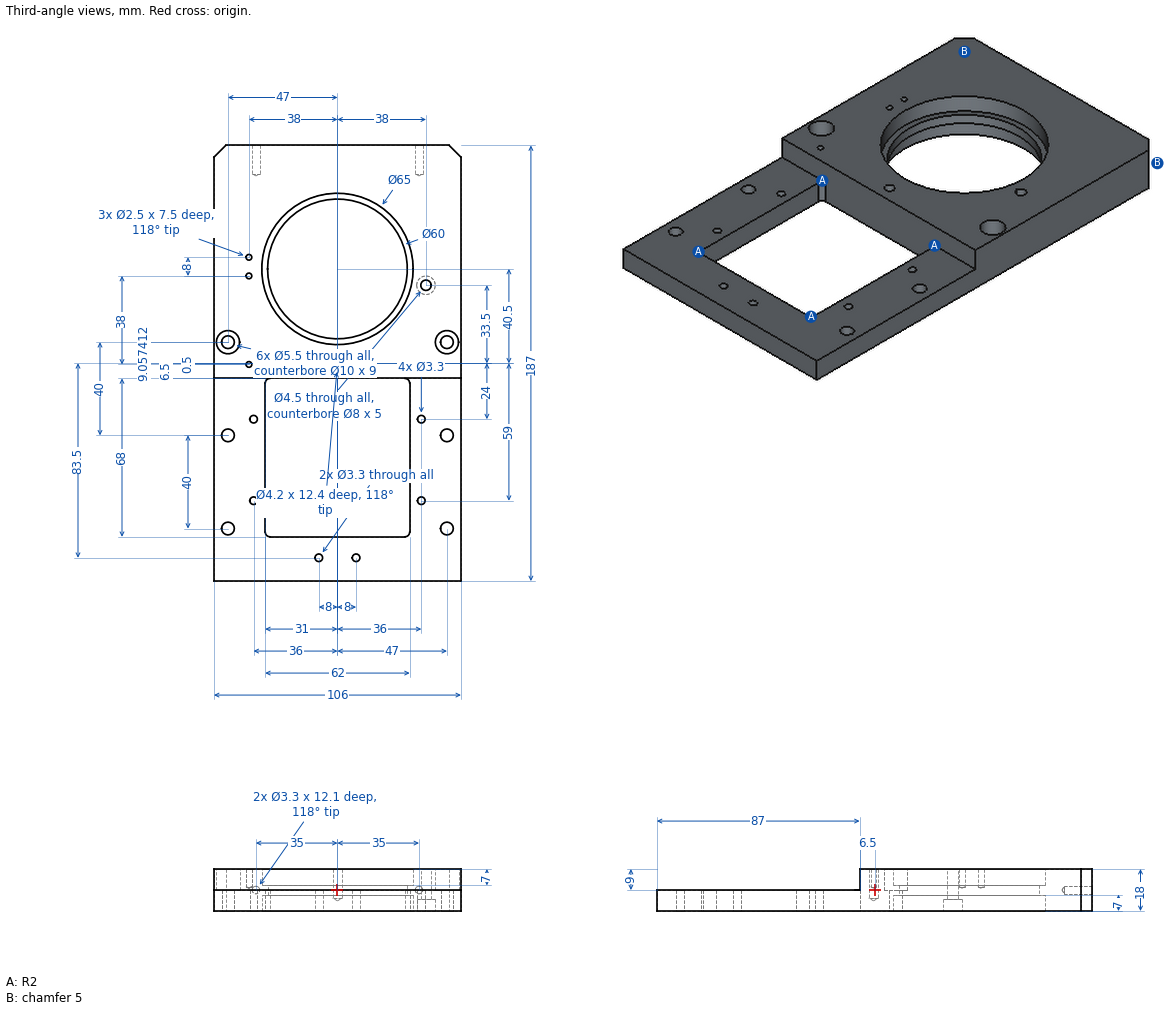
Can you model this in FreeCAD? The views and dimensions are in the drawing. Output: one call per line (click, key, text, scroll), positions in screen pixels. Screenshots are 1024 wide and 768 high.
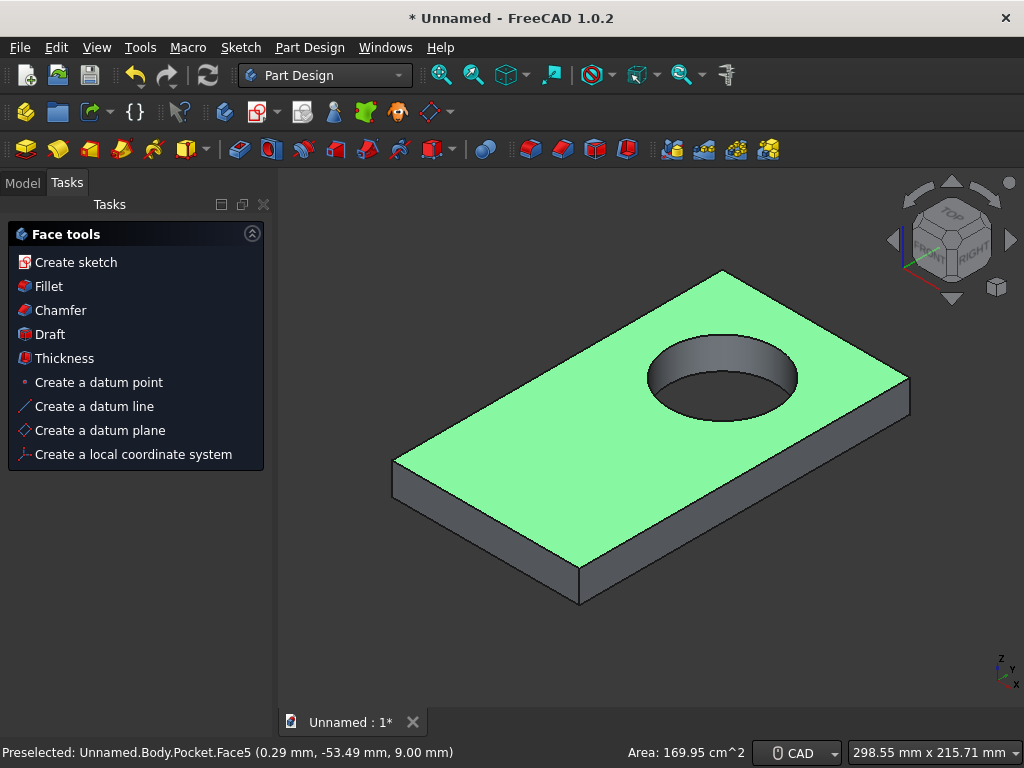
click(258, 112)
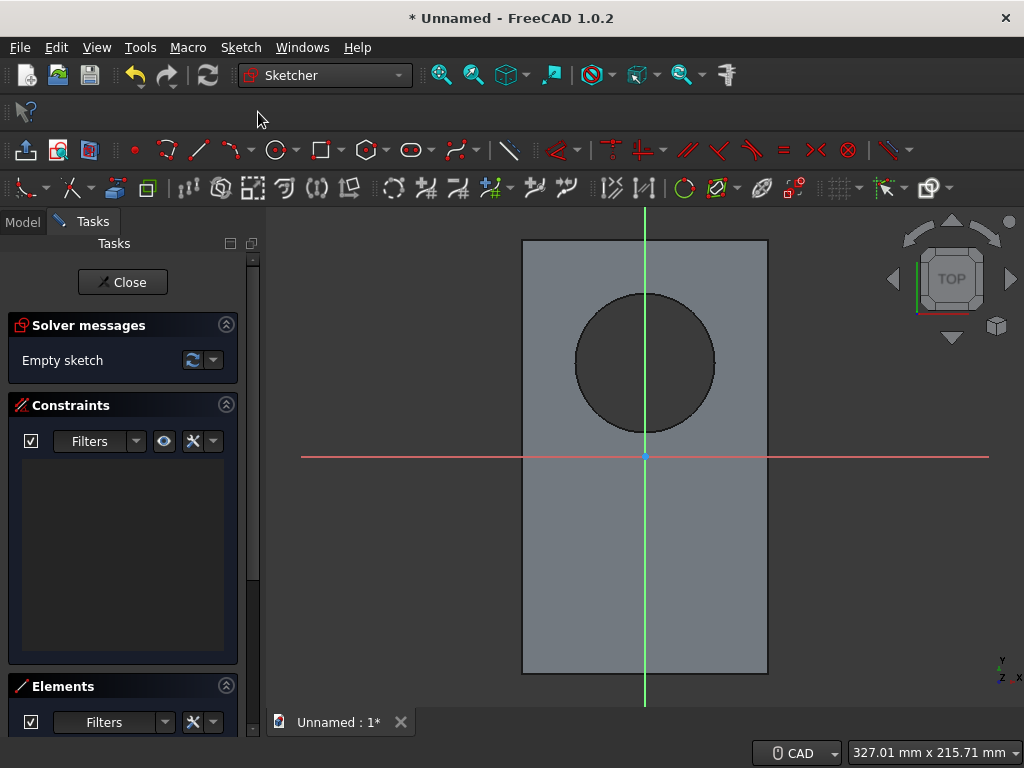
scroll(728, 269, up, 3)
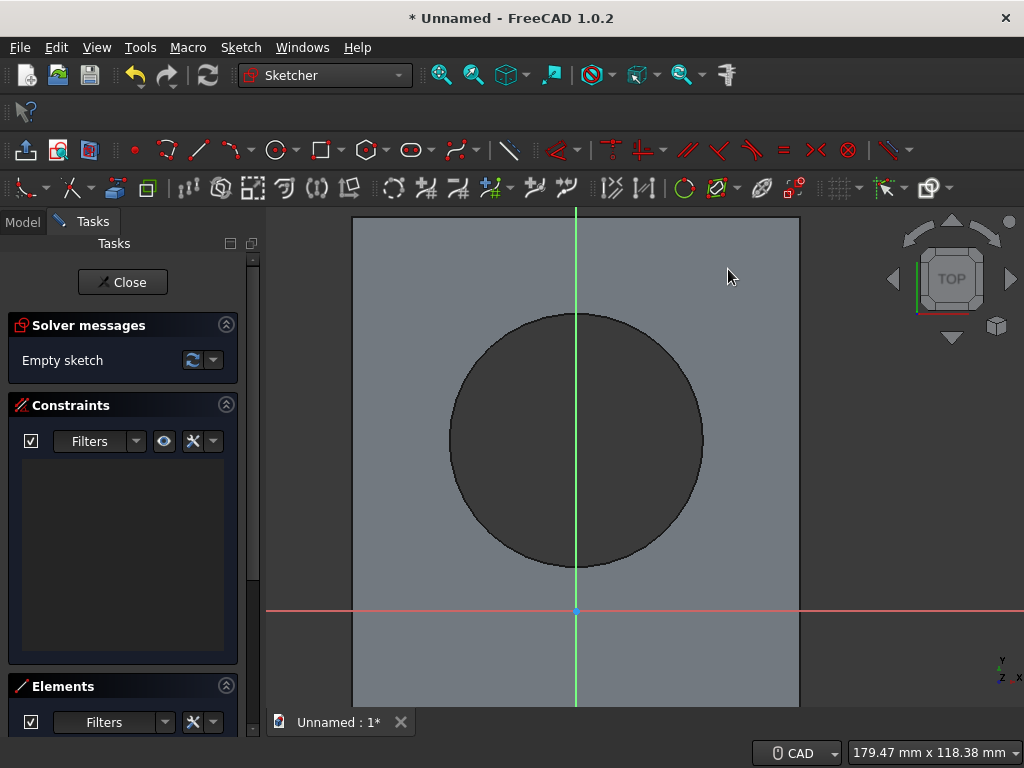
click(276, 150)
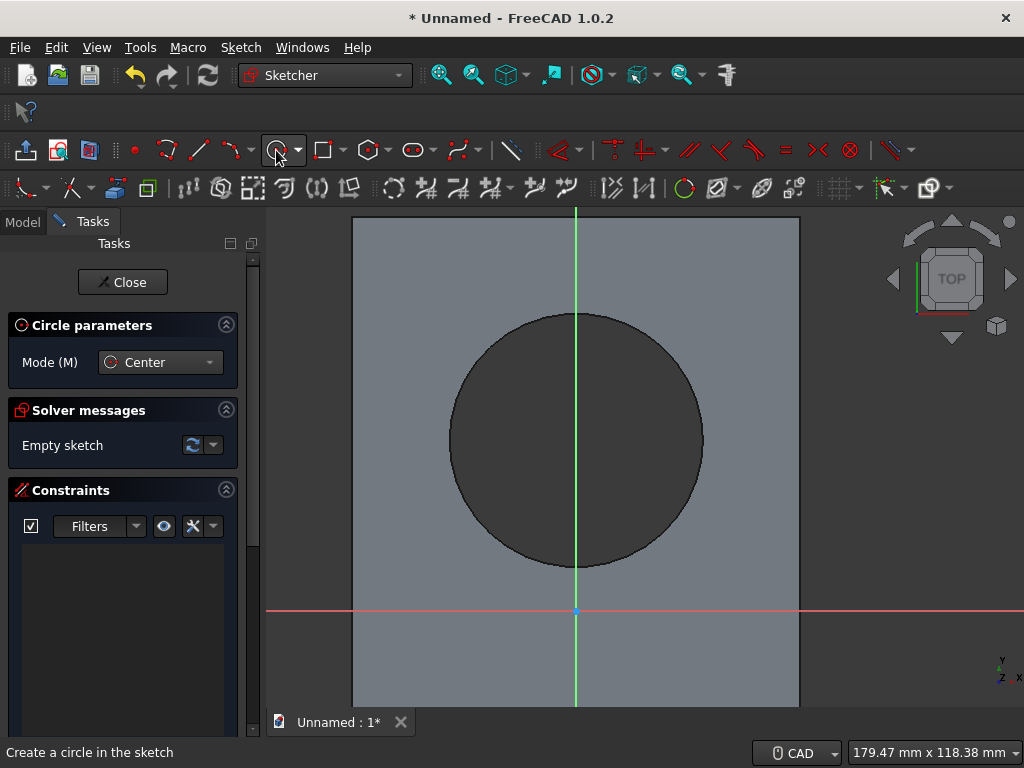
click(576, 440)
click(673, 343)
key(Escape)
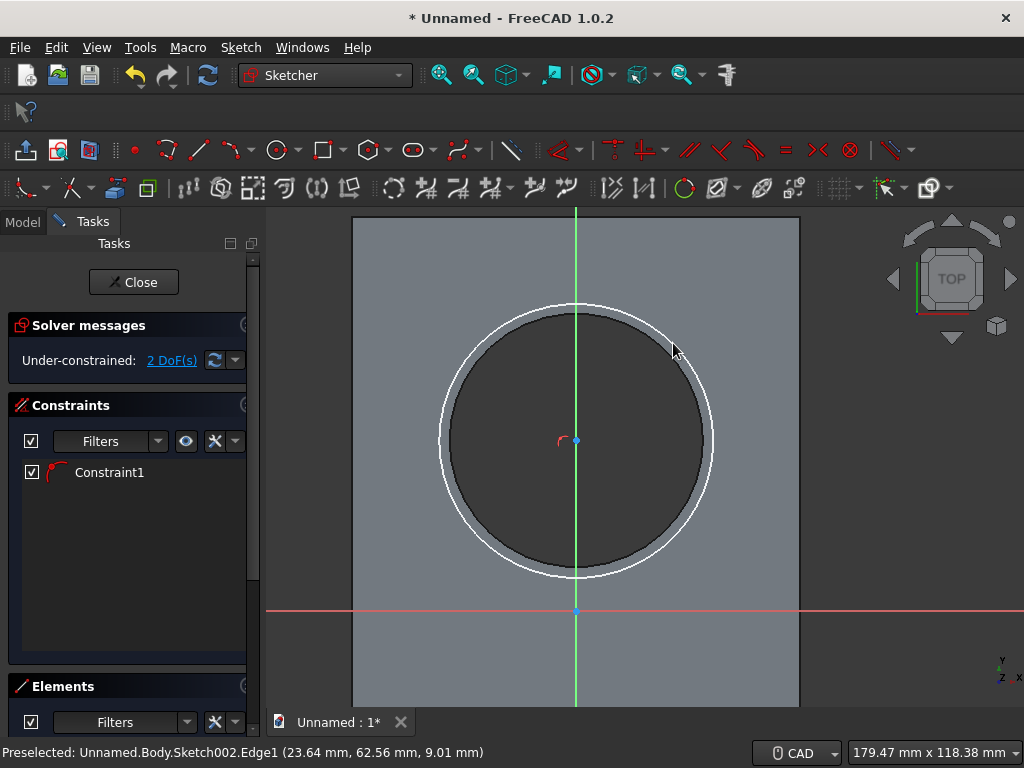
click(558, 150)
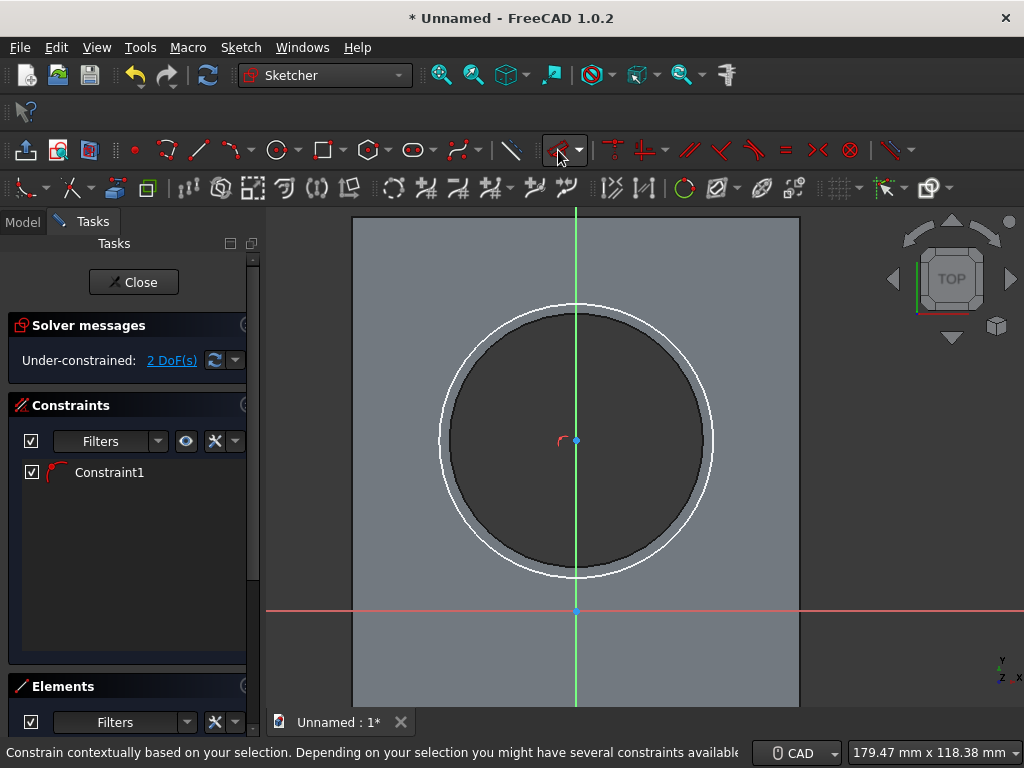
click(673, 344)
click(696, 321)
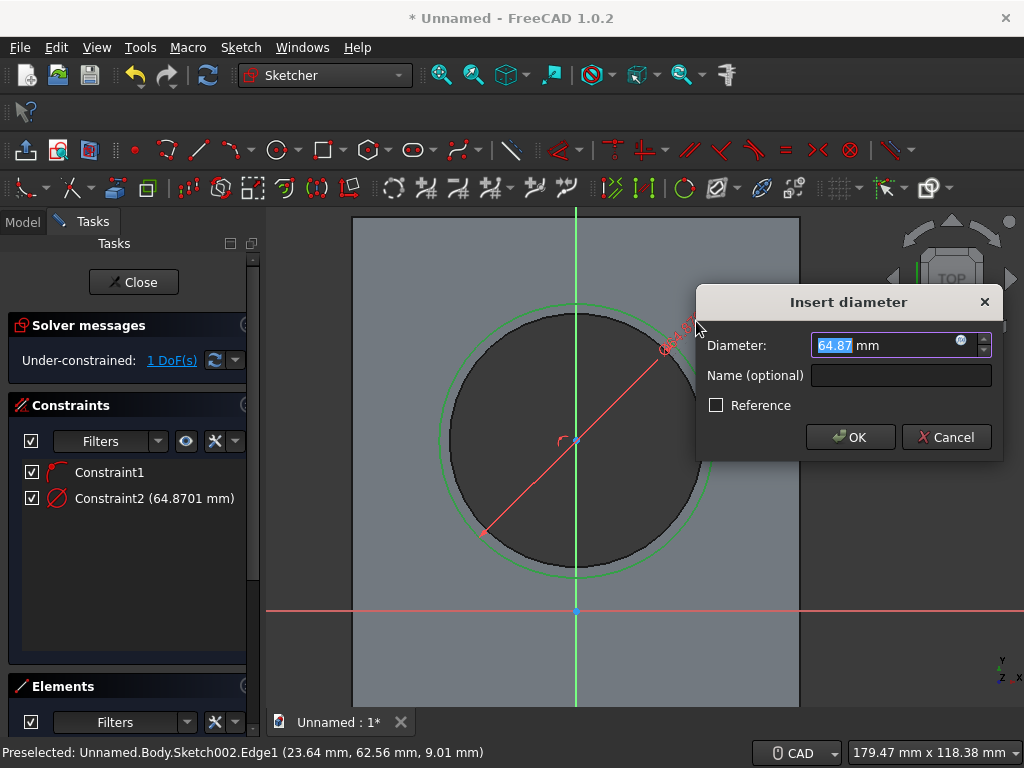
text(65)
key(Return)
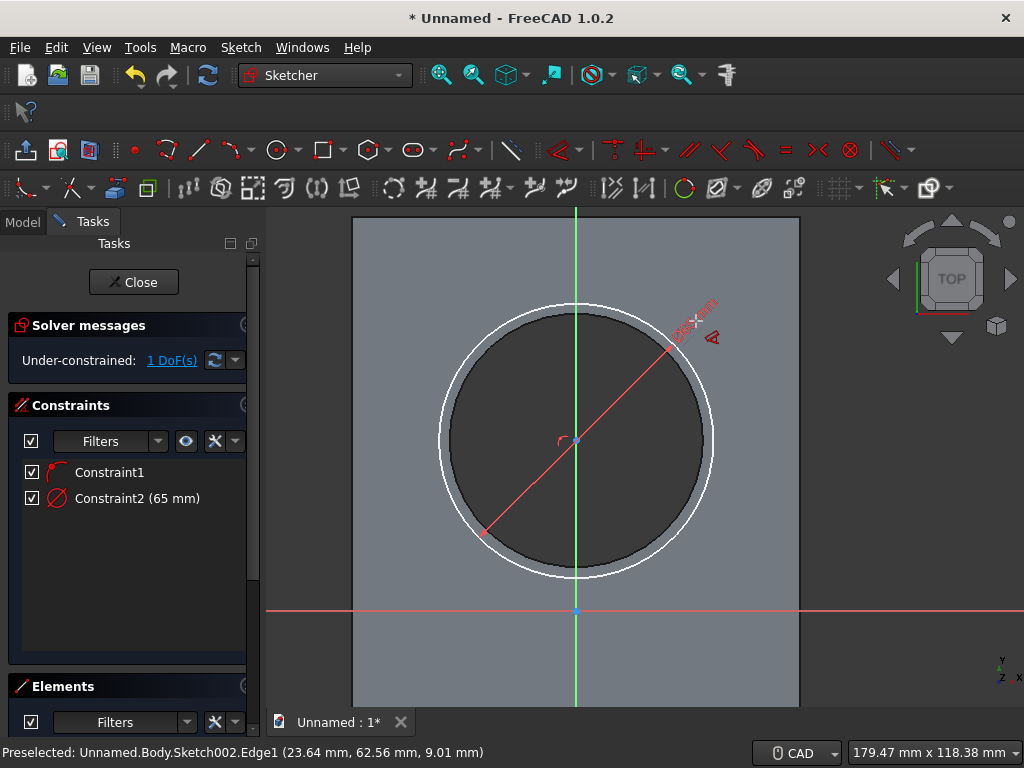
click(576, 441)
click(610, 526)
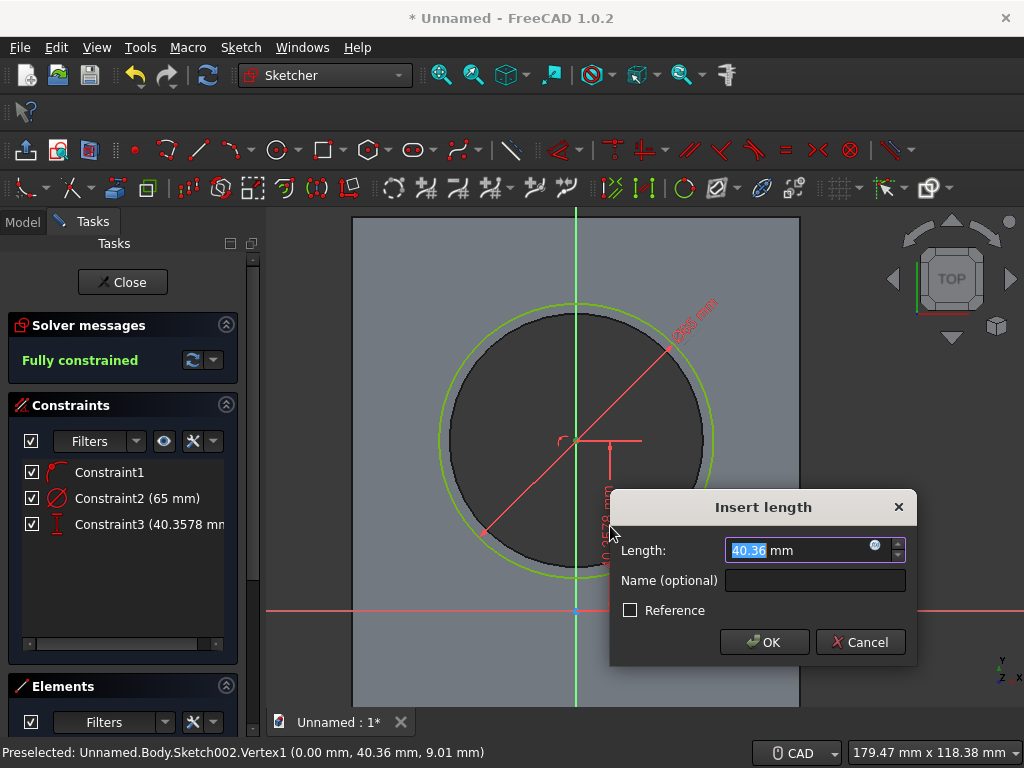
text(40.5)
key(Return)
key(Escape)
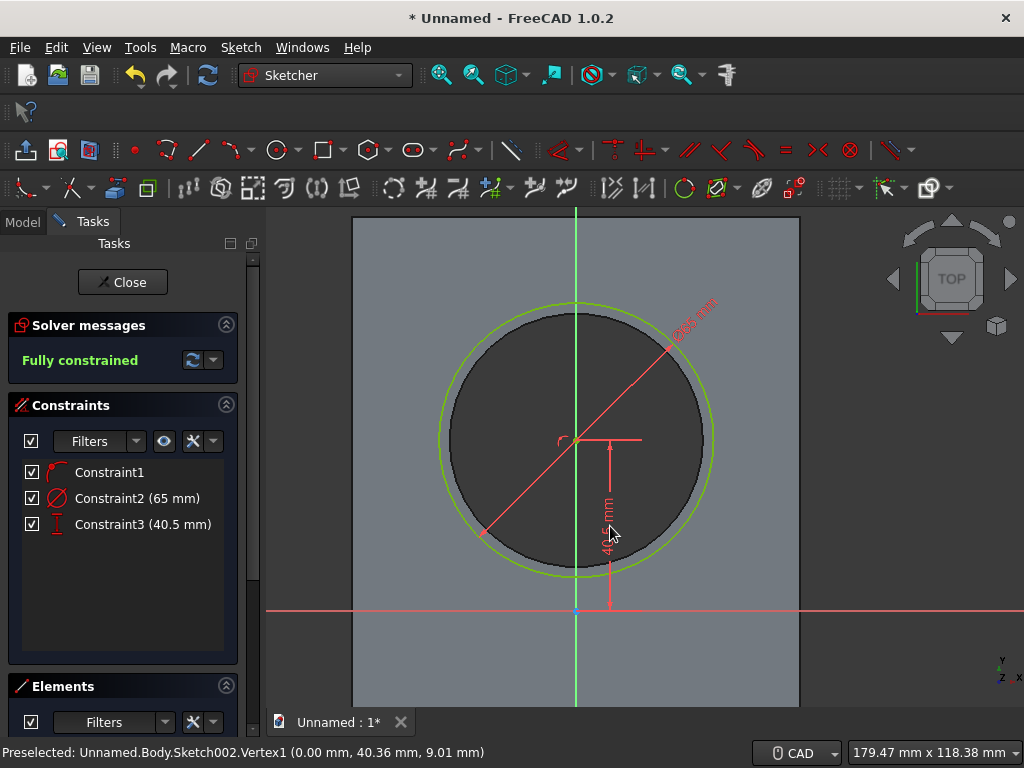
click(123, 282)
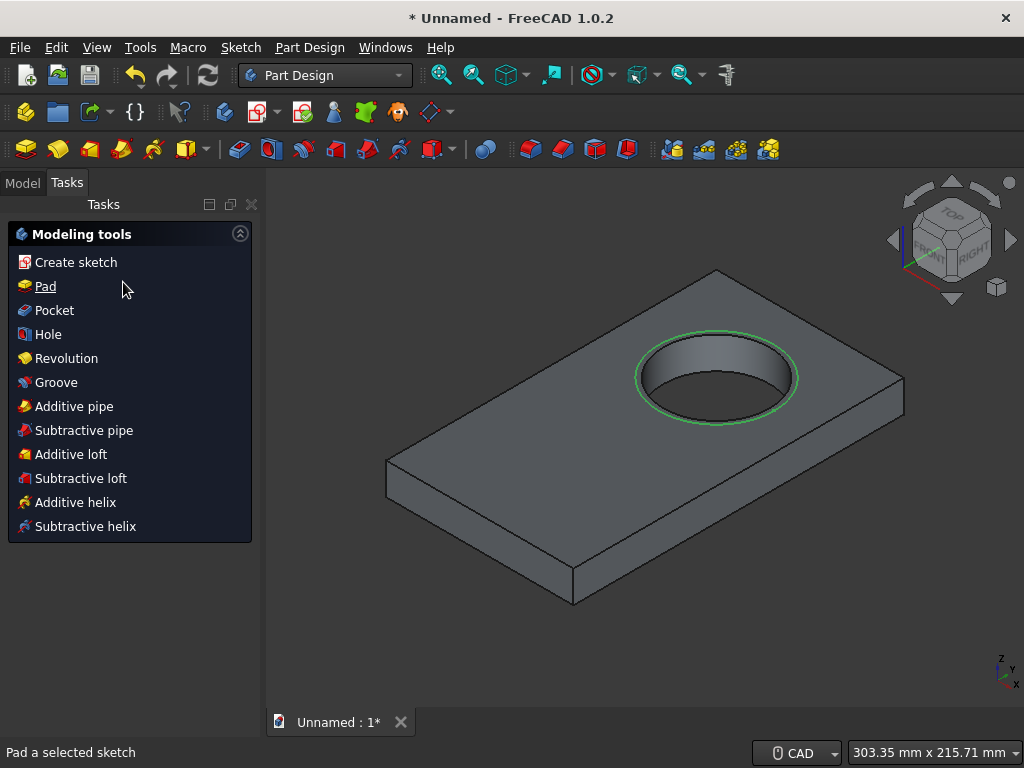
click(240, 150)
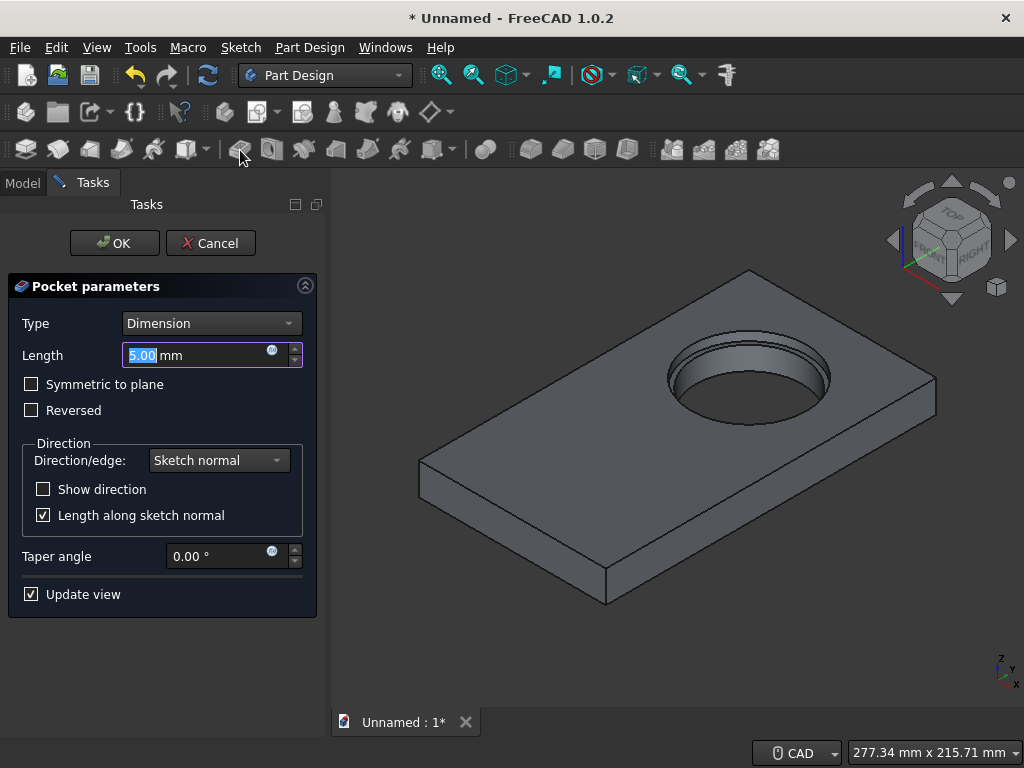
text(7)
key(Tab)